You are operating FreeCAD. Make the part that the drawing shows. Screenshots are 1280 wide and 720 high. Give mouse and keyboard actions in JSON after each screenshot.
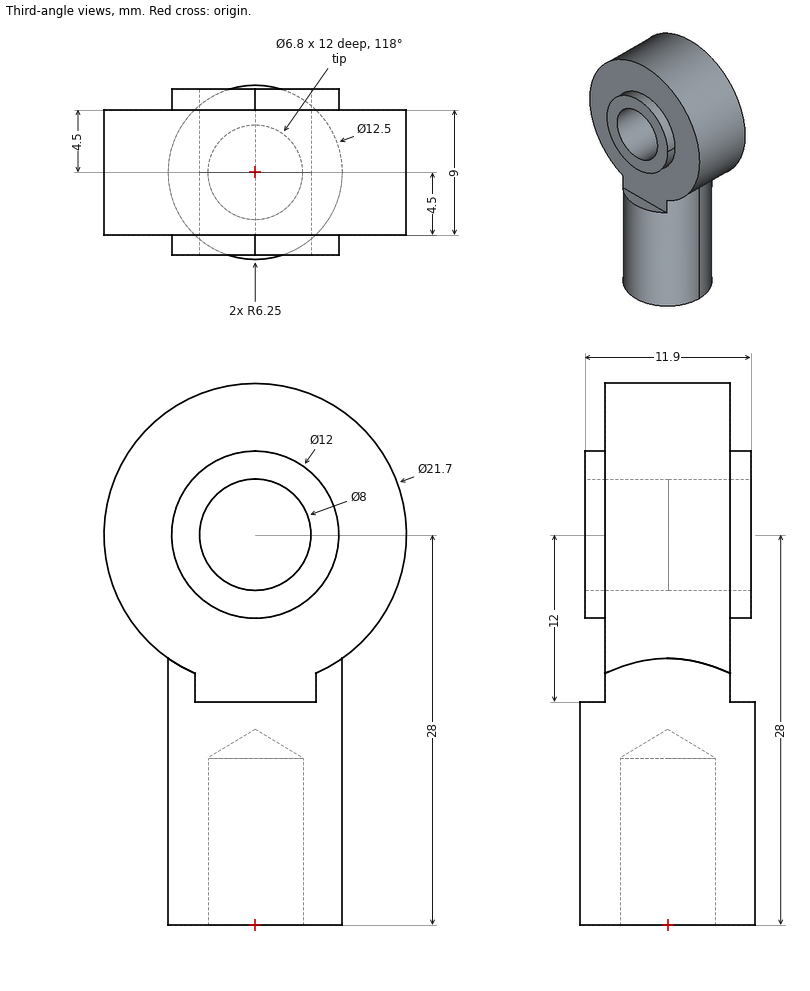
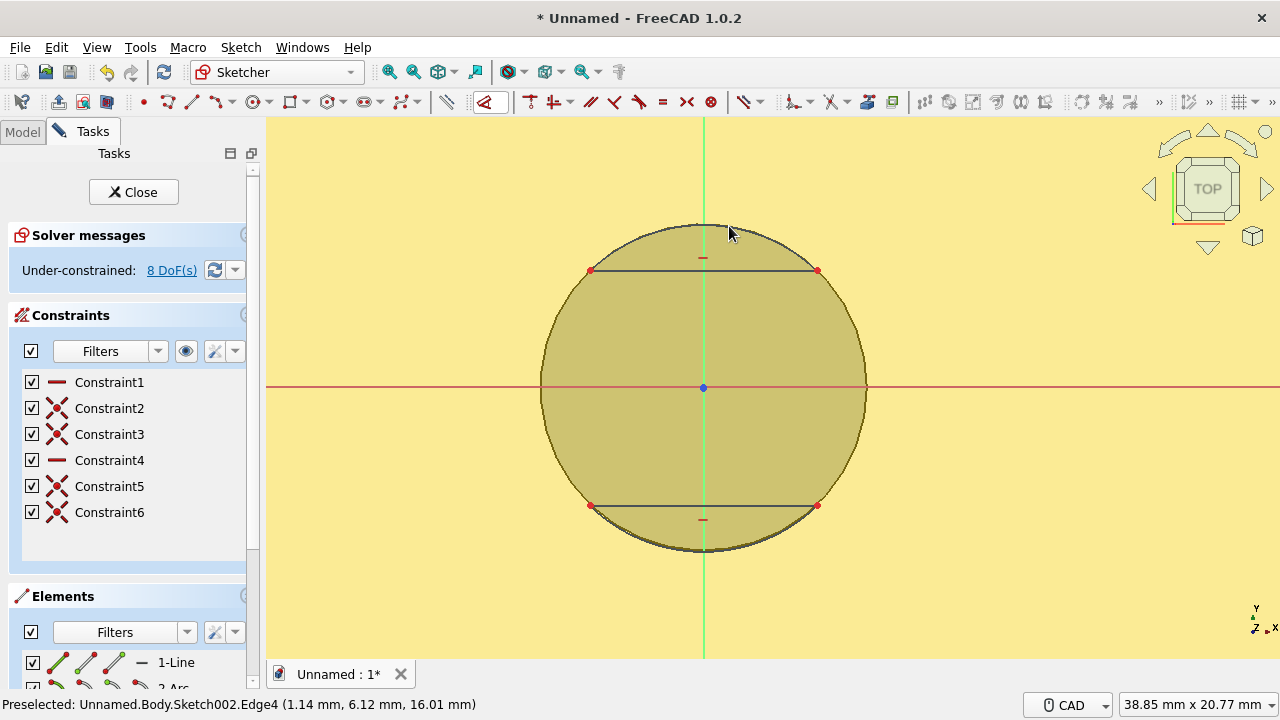
{"action": "left_click", "coordinate": [654, 544]}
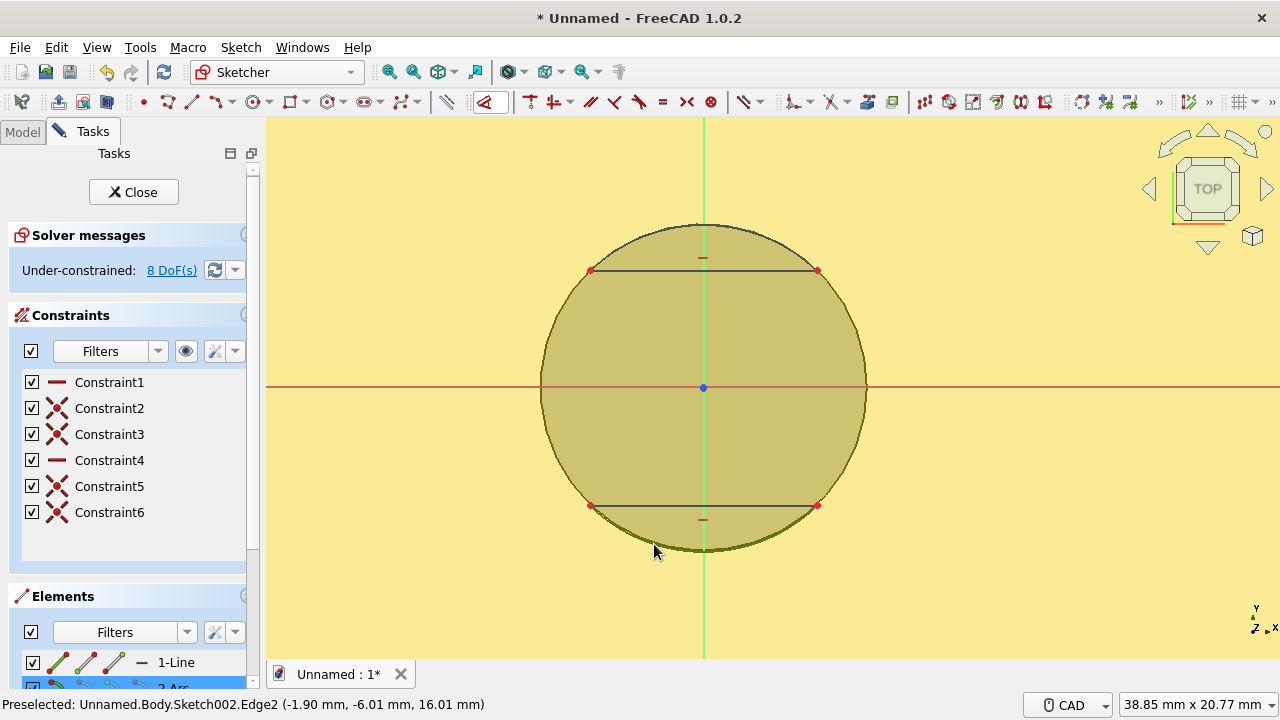
{"action": "left_click", "coordinate": [753, 233]}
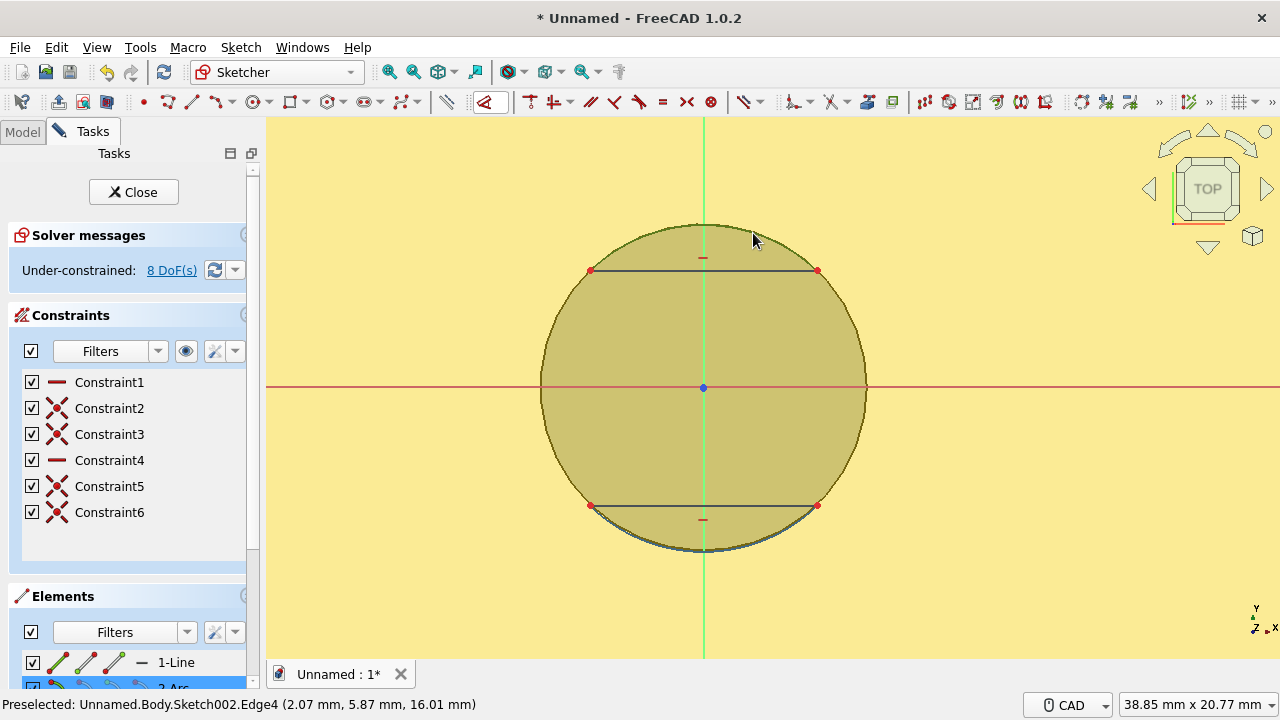
{"action": "key", "text": "c"}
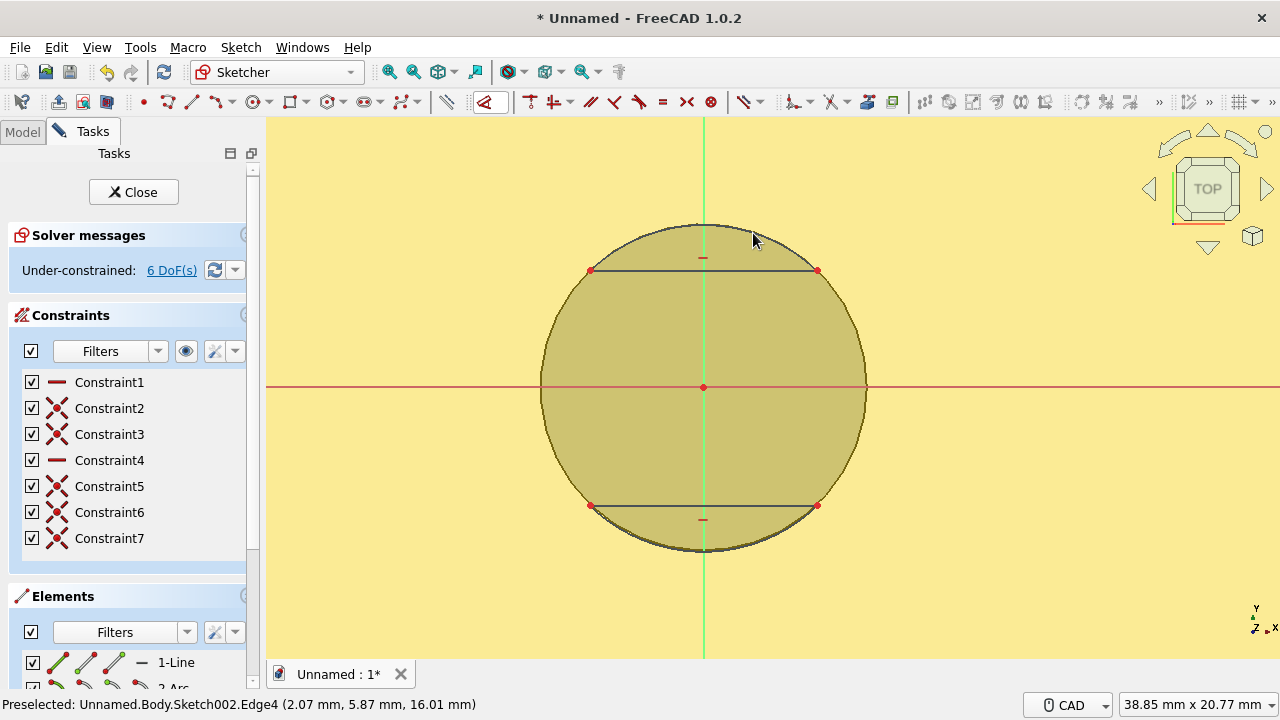
{"action": "left_click_drag", "start_coordinate": [694, 377], "coordinate": [714, 398]}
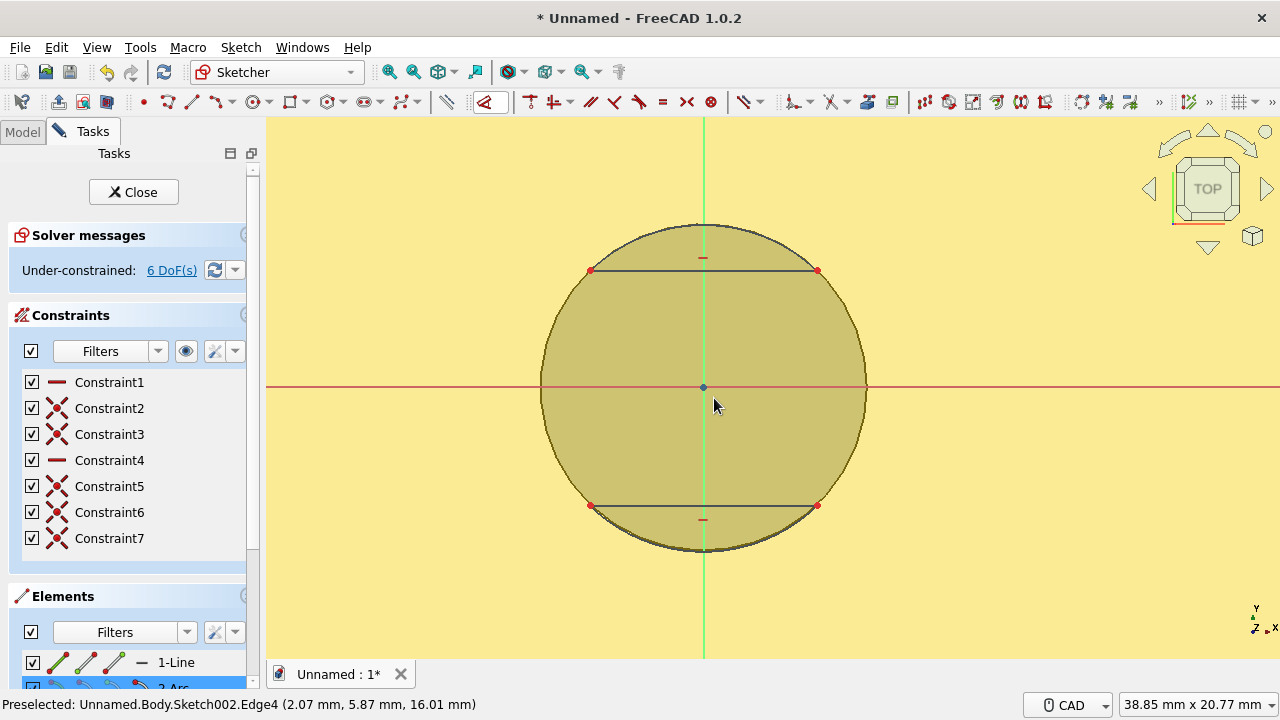
{"action": "left_click", "coordinate": [530, 102]}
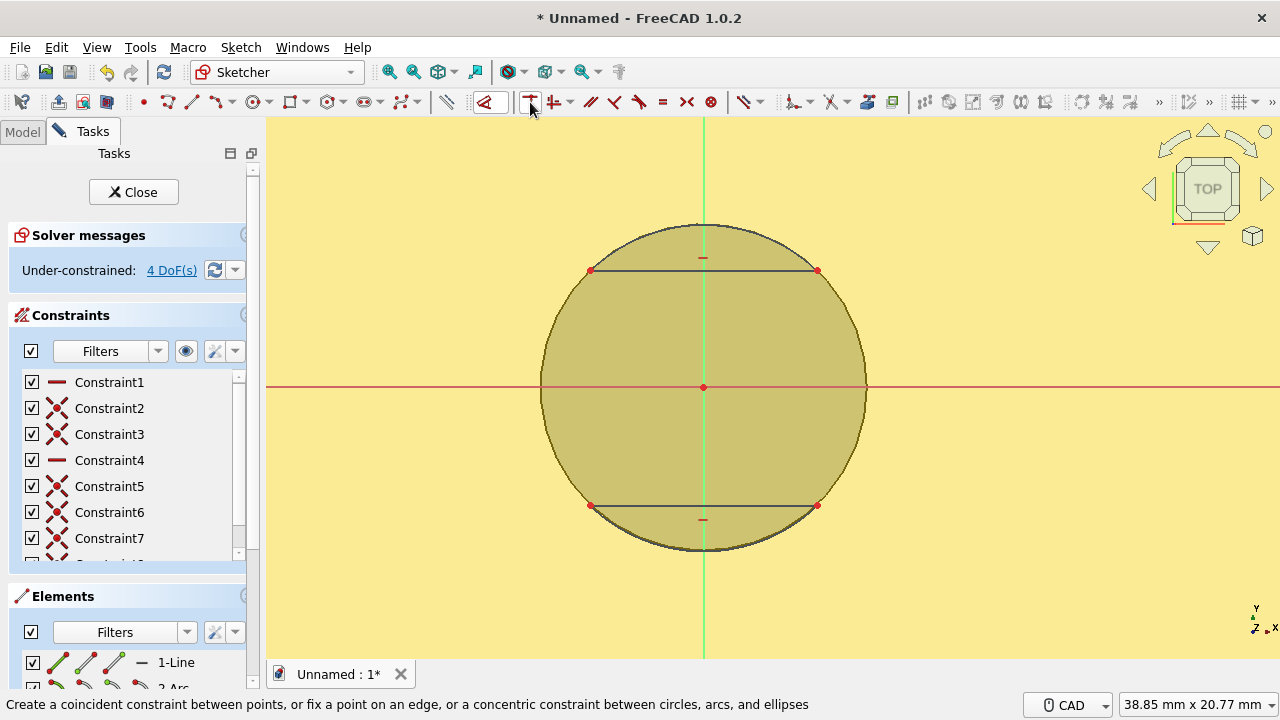
{"action": "left_click", "coordinate": [654, 544]}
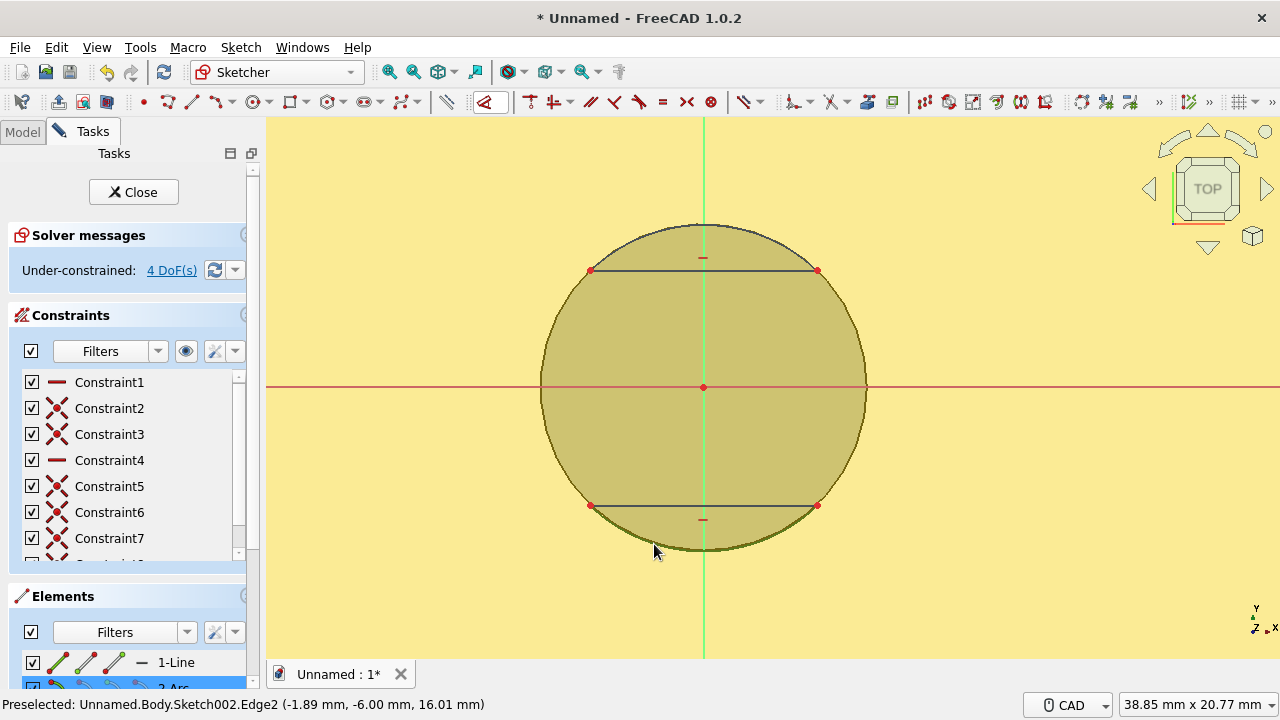
{"action": "left_click", "coordinate": [753, 233]}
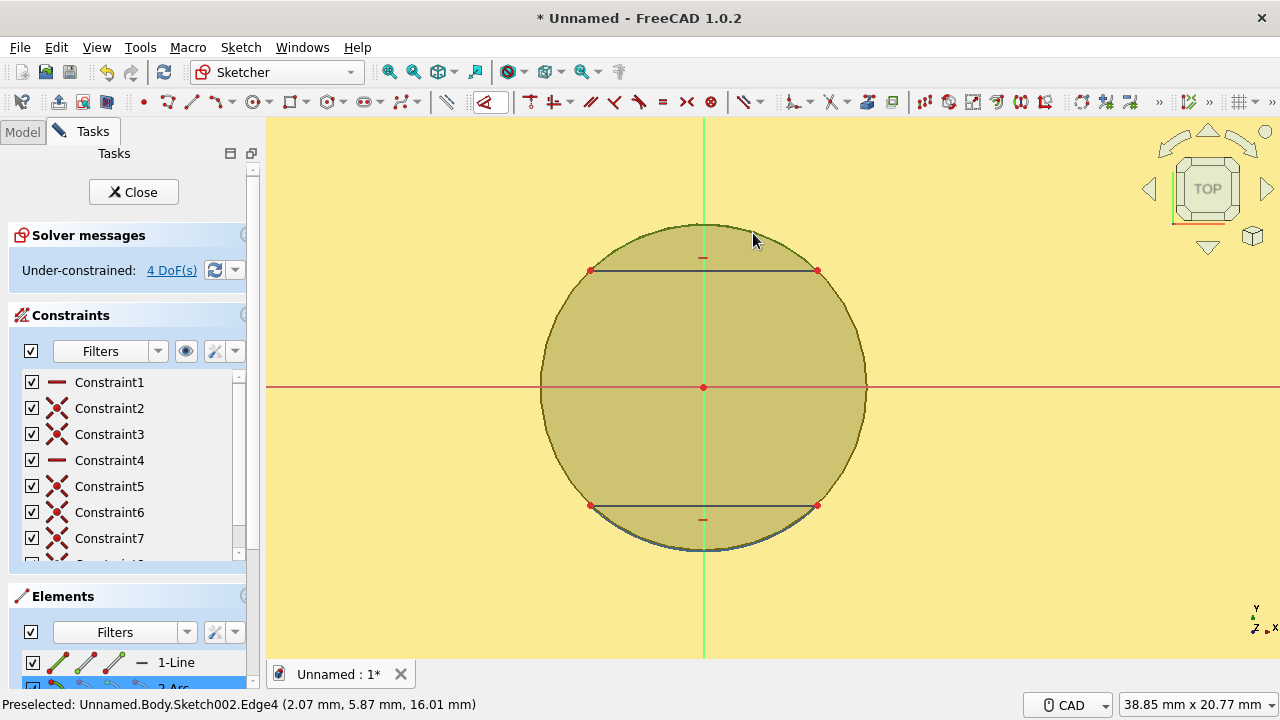
{"action": "left_click", "coordinate": [664, 102]}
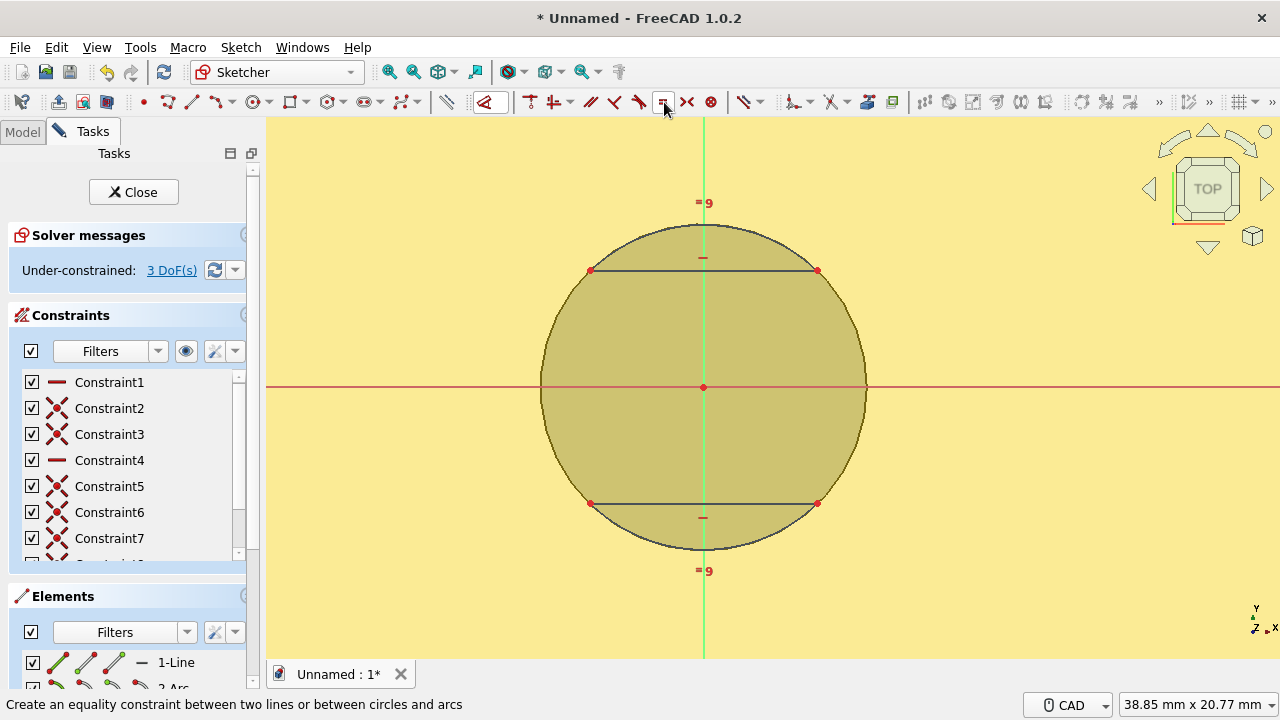
{"action": "left_click", "coordinate": [654, 542]}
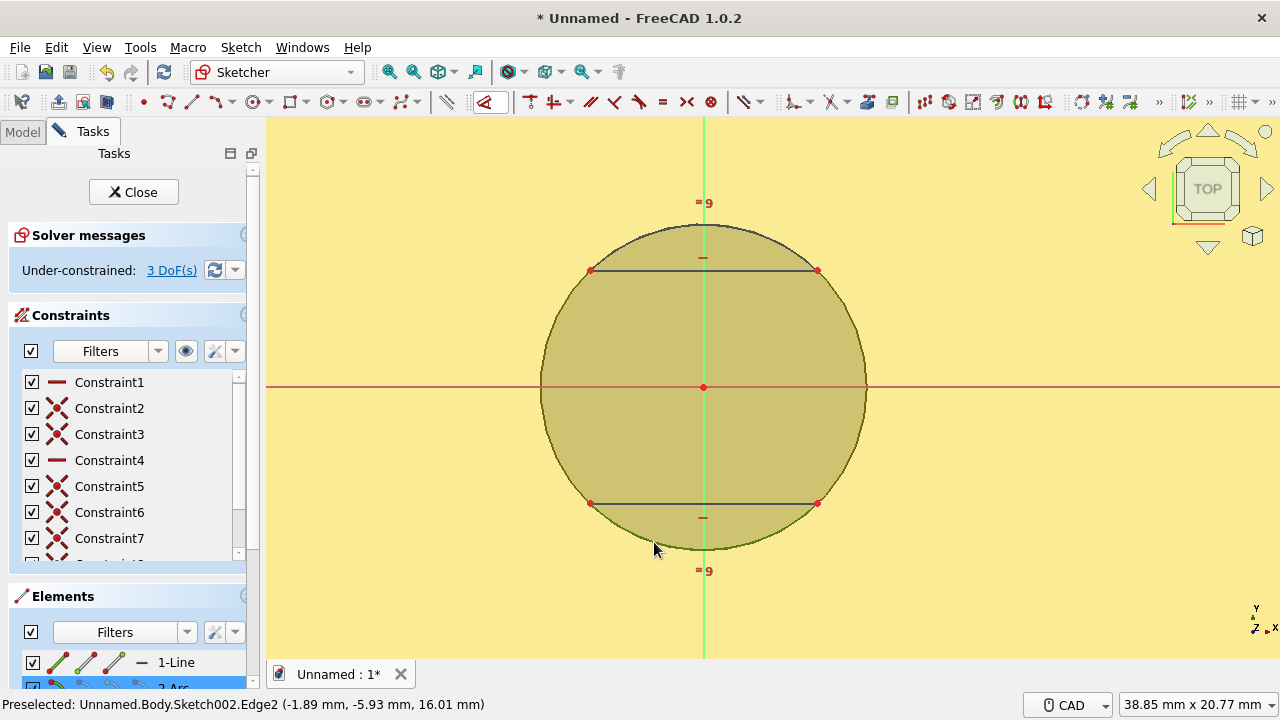
{"action": "key", "text": "k r"}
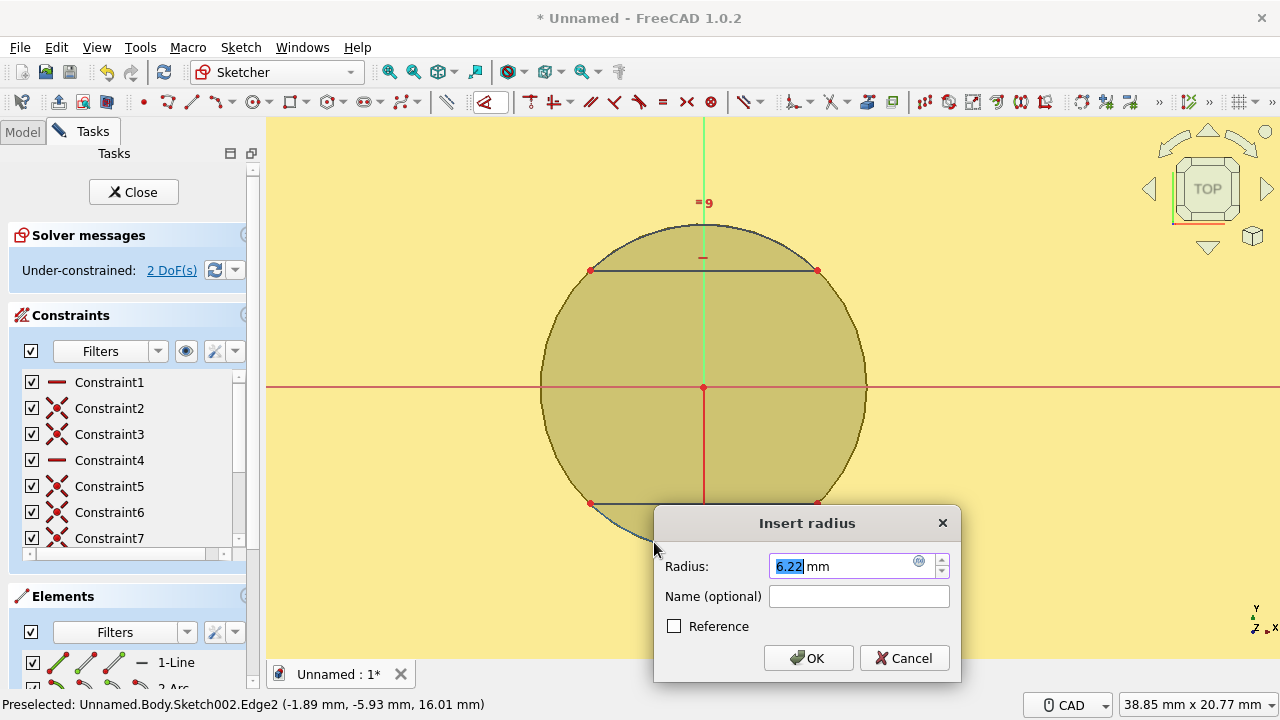
{"action": "type", "text": "6.25"}
{"action": "key", "text": "Return"}